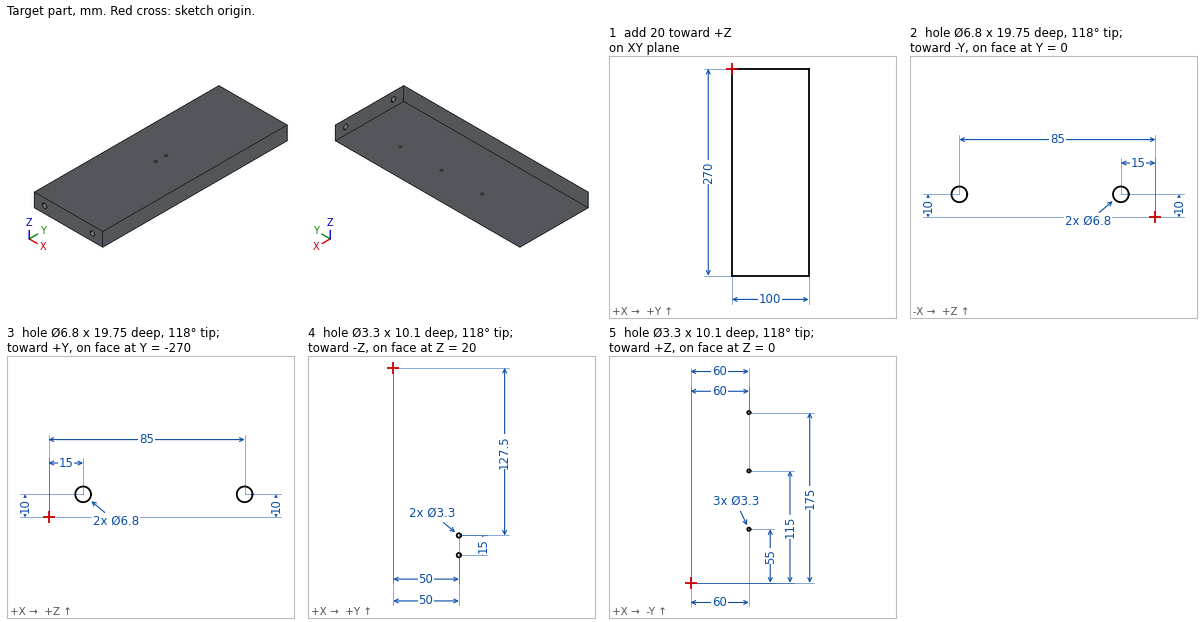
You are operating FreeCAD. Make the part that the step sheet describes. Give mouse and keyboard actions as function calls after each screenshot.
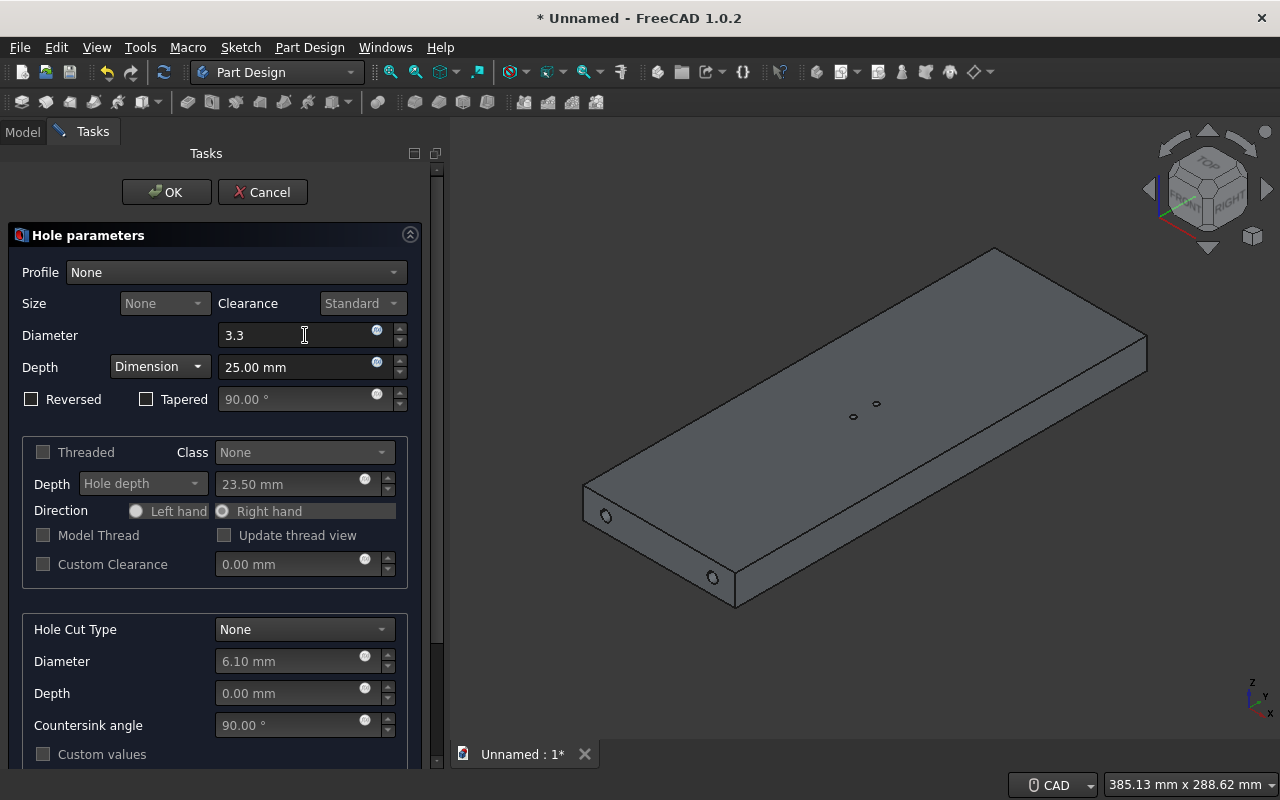
triple_click(305, 367)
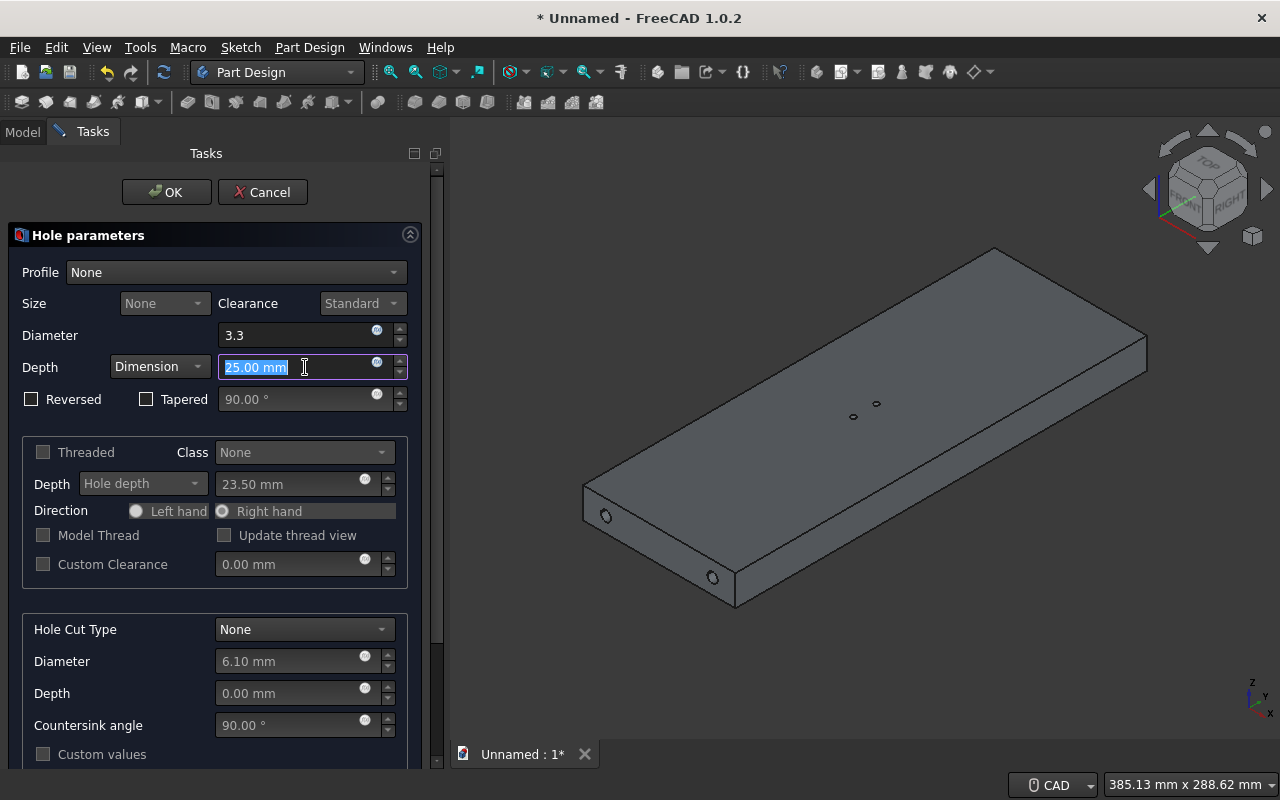
text(10.1)
key(Tab)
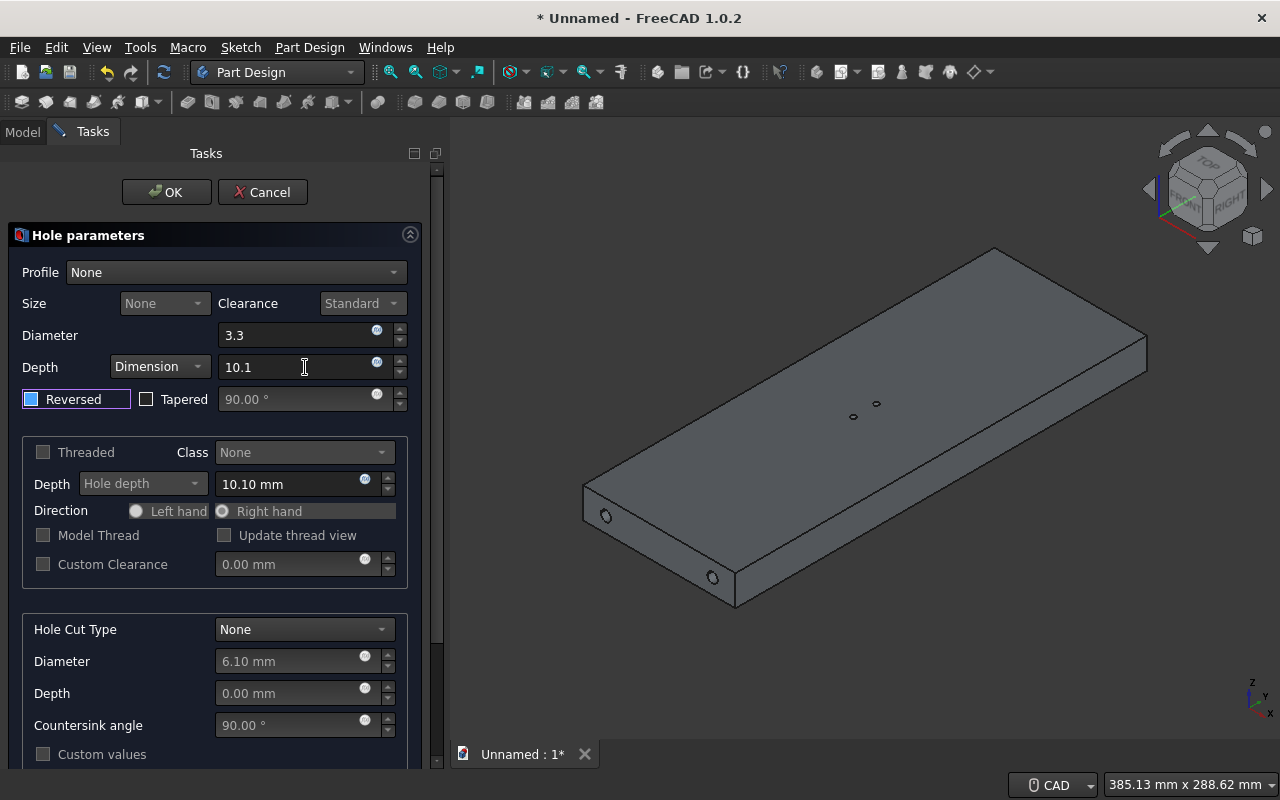
click(167, 192)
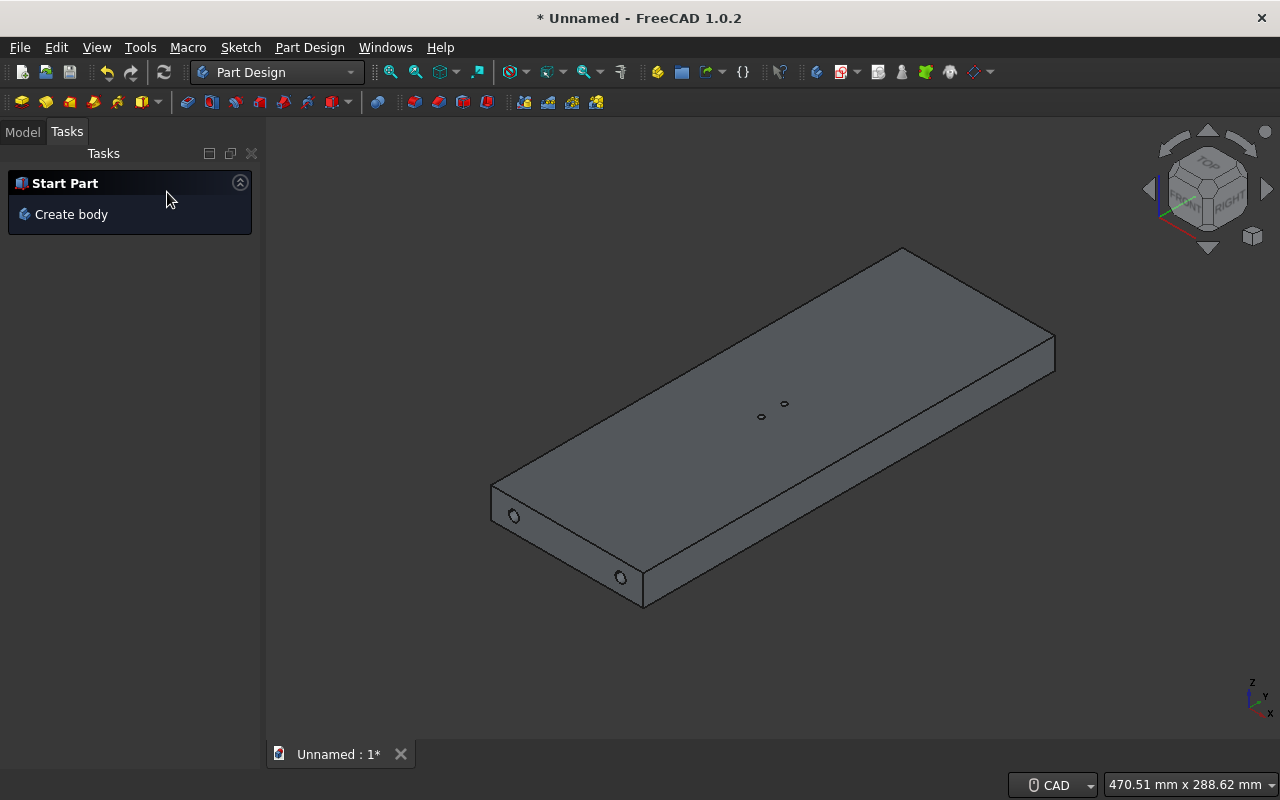
key(5)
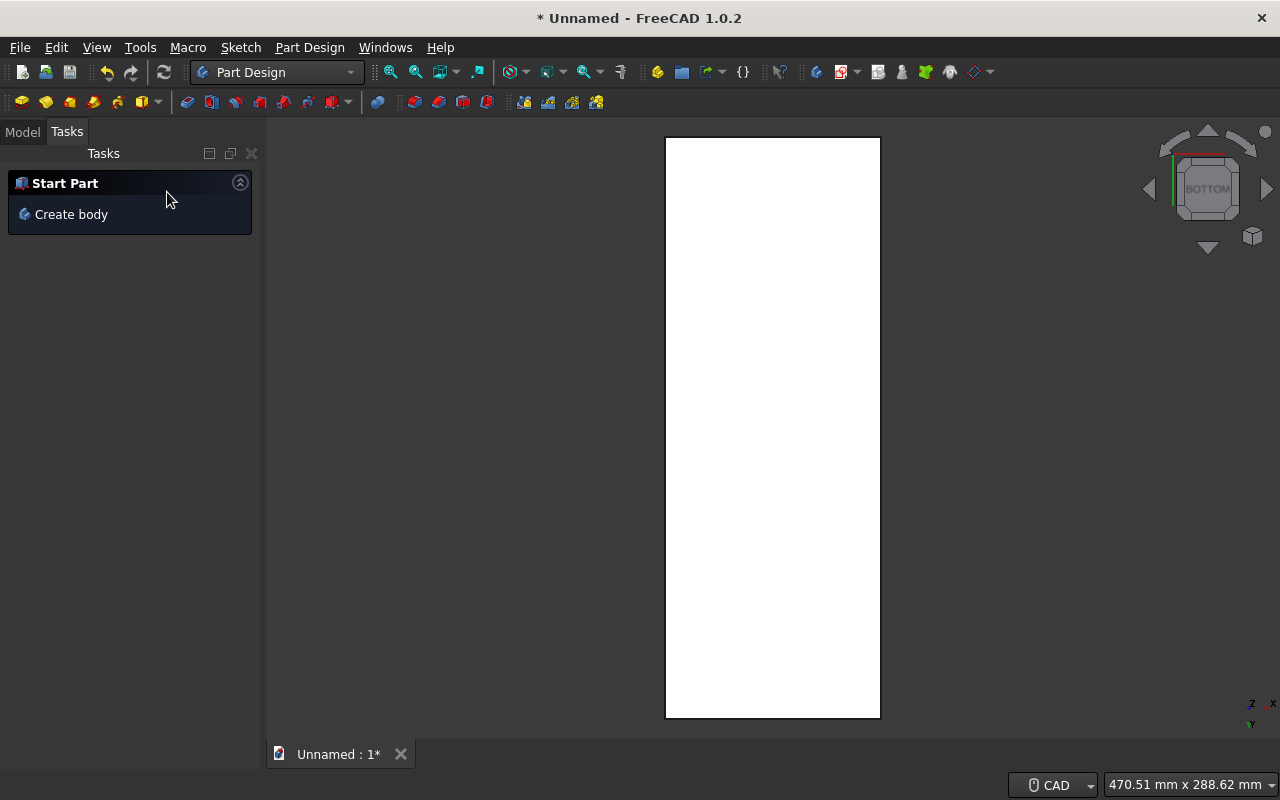
click(773, 593)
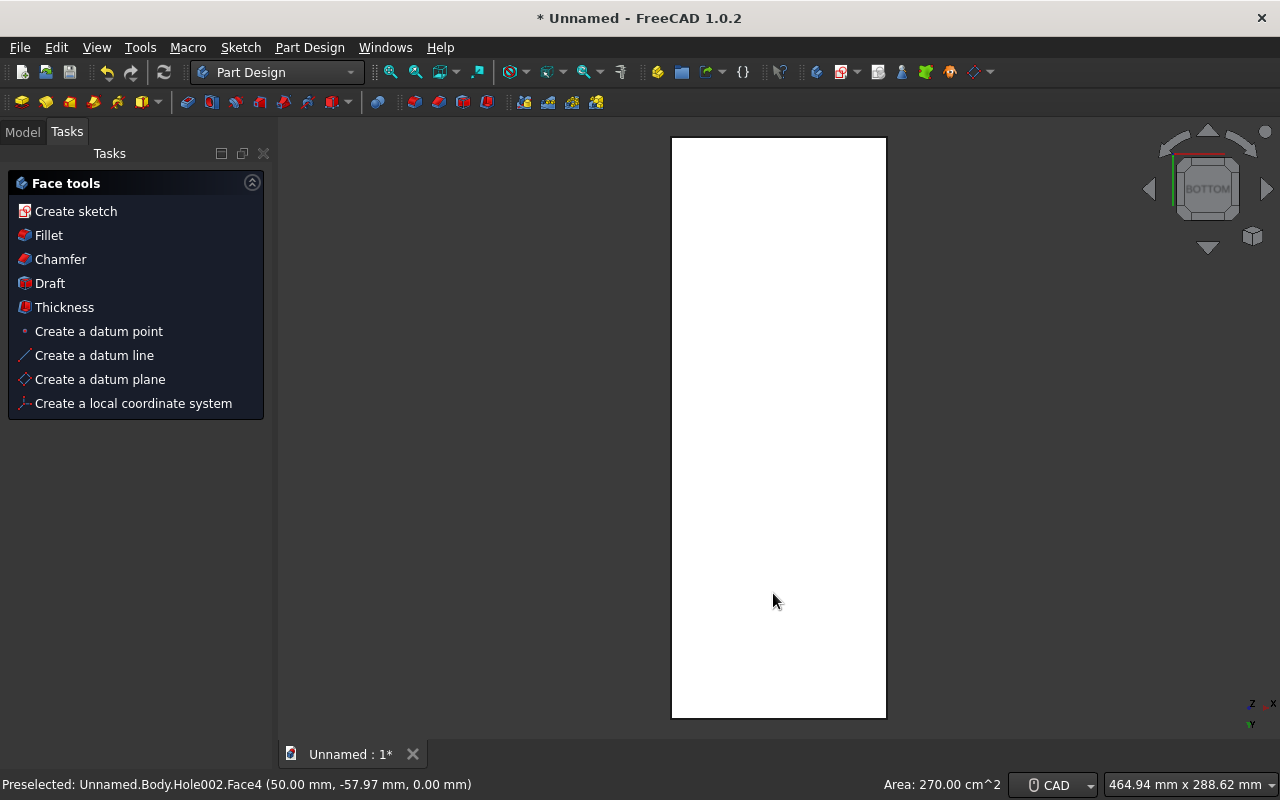
click(842, 72)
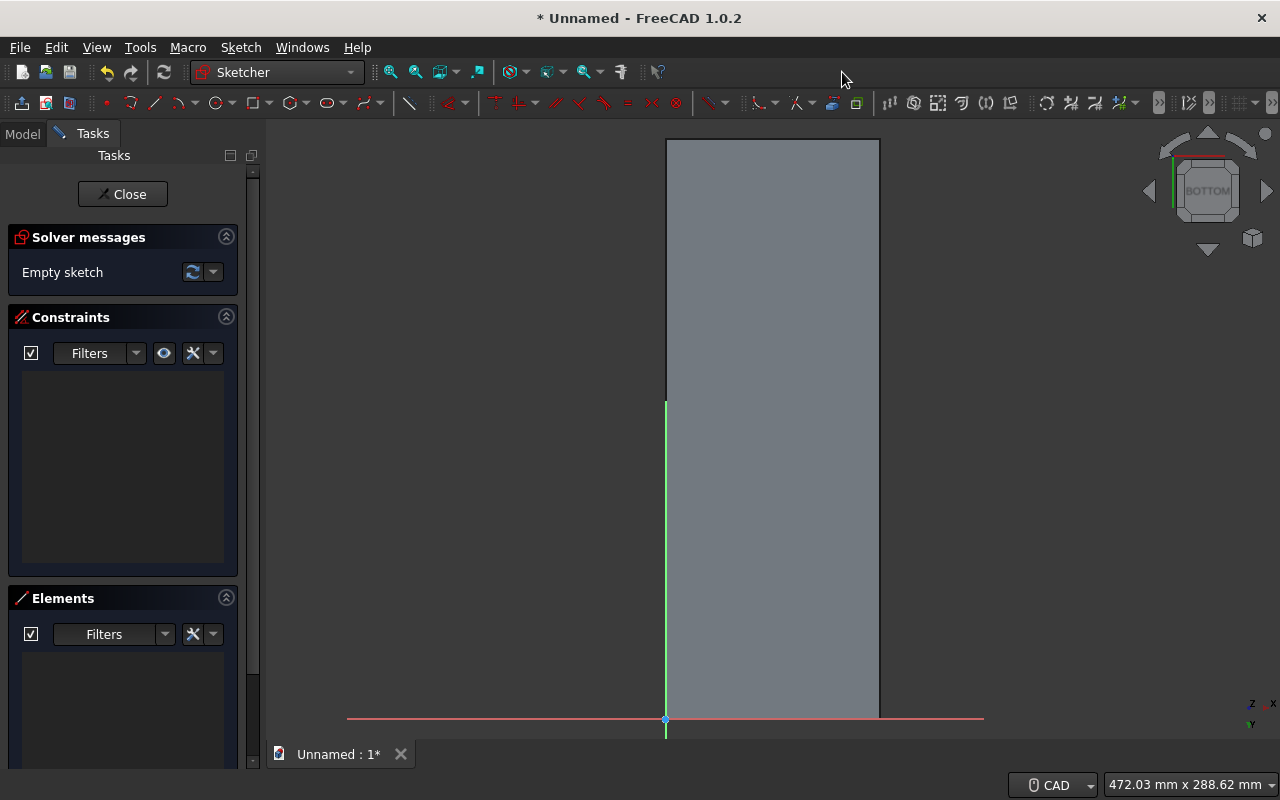
scroll(581, 147, down, 1)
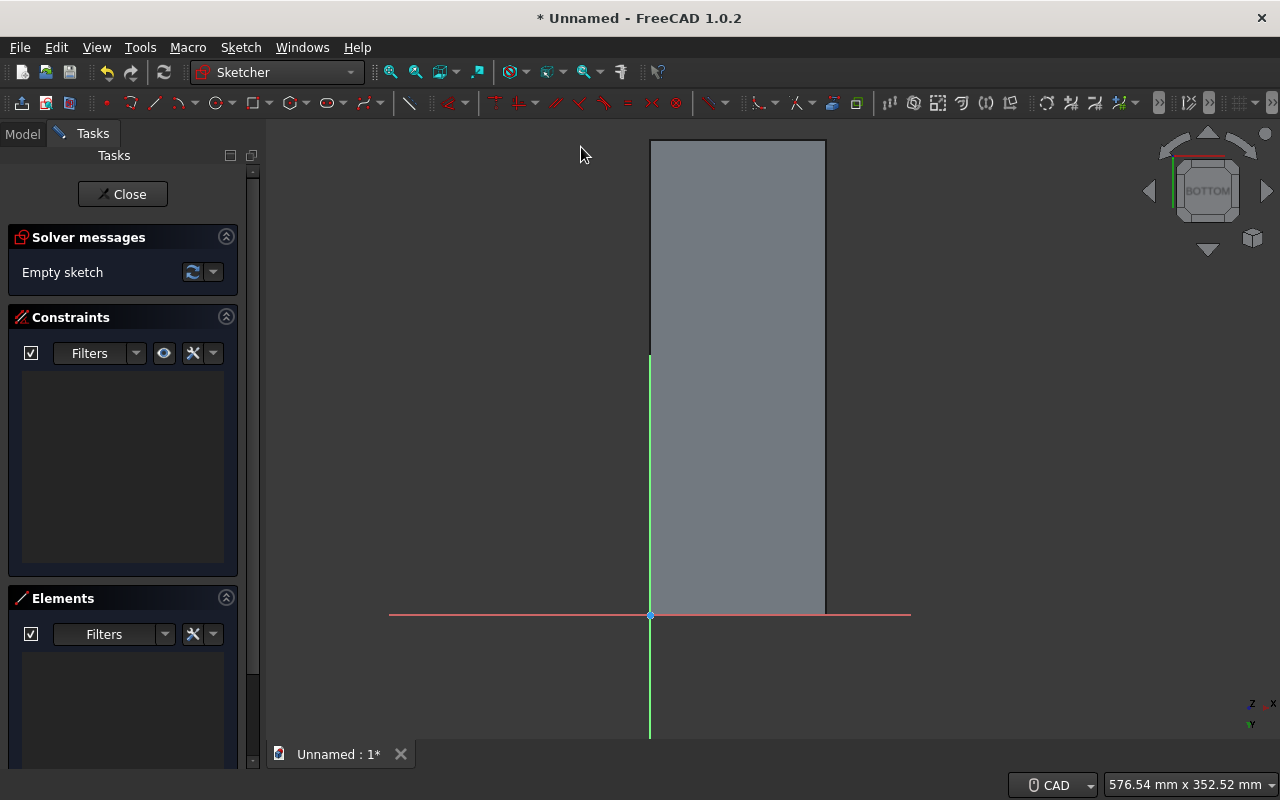
key(g)
key(c)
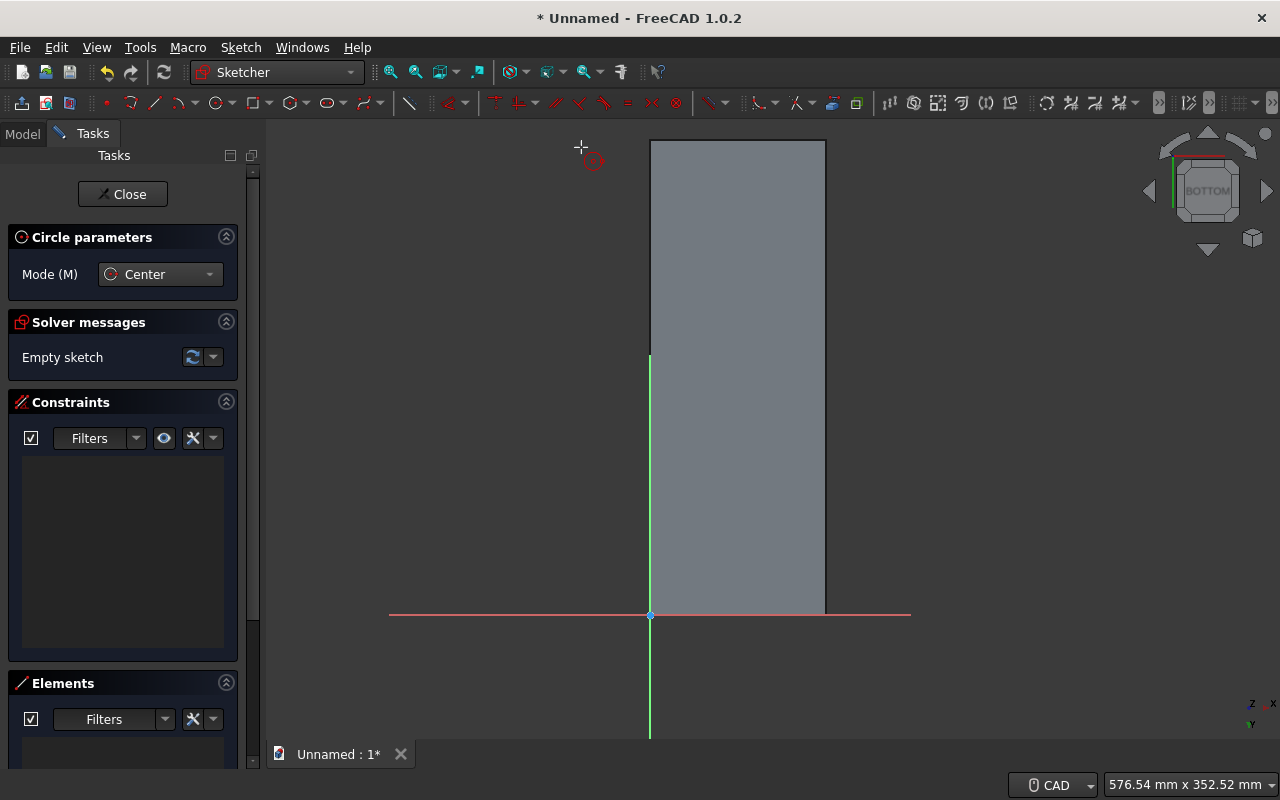
scroll(756, 519, up, 11)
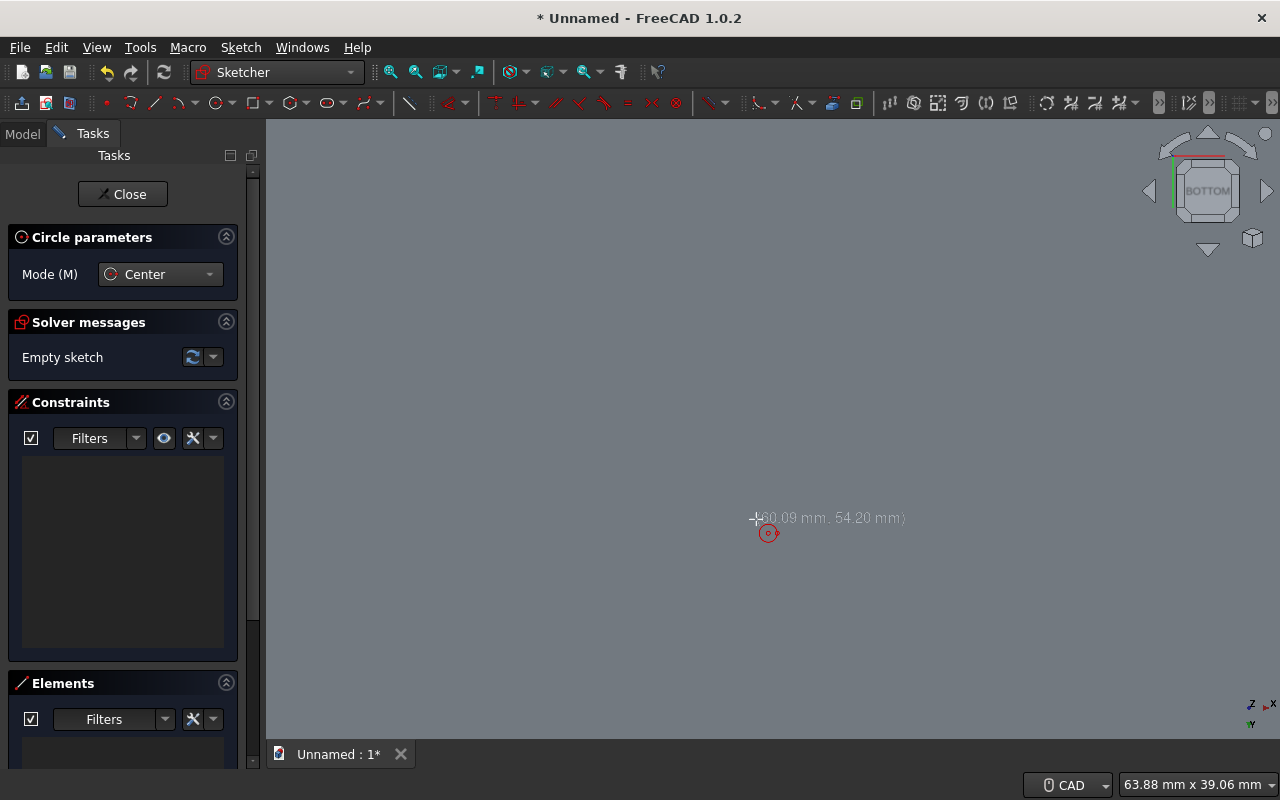
scroll(770, 499, down, 10)